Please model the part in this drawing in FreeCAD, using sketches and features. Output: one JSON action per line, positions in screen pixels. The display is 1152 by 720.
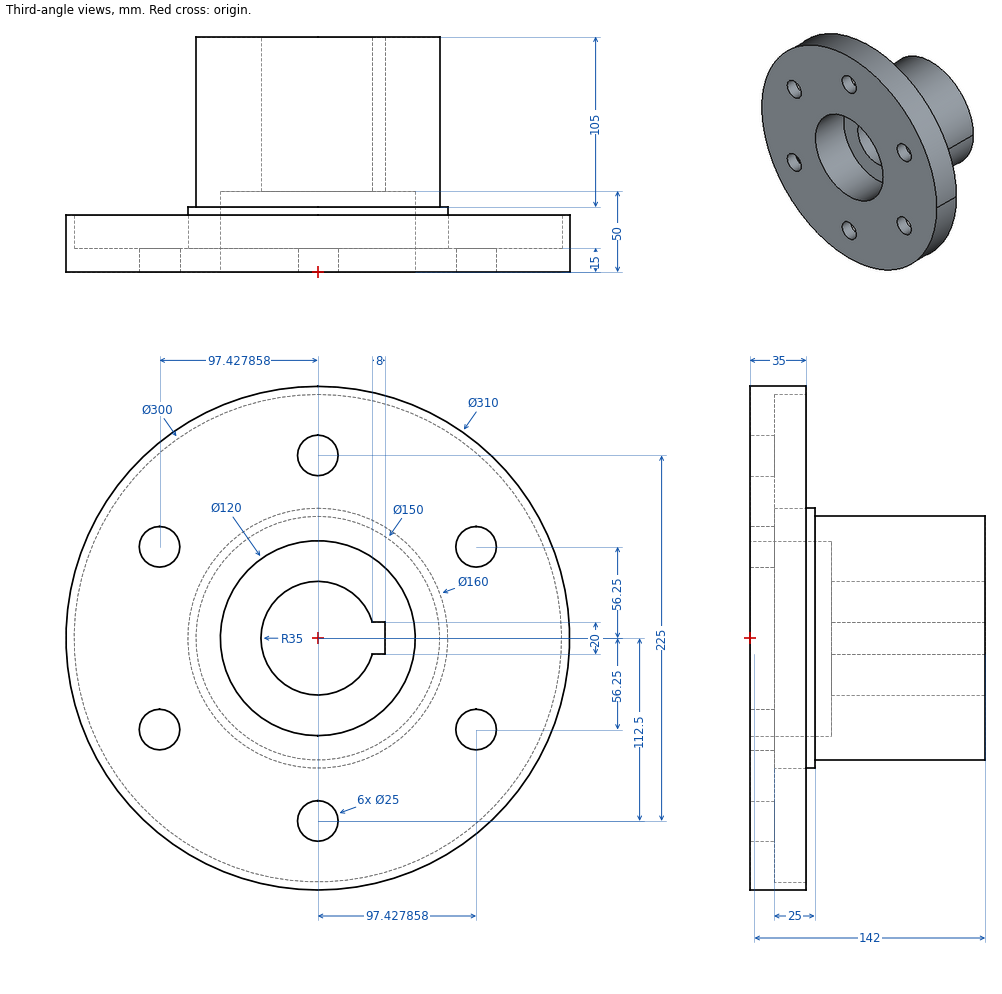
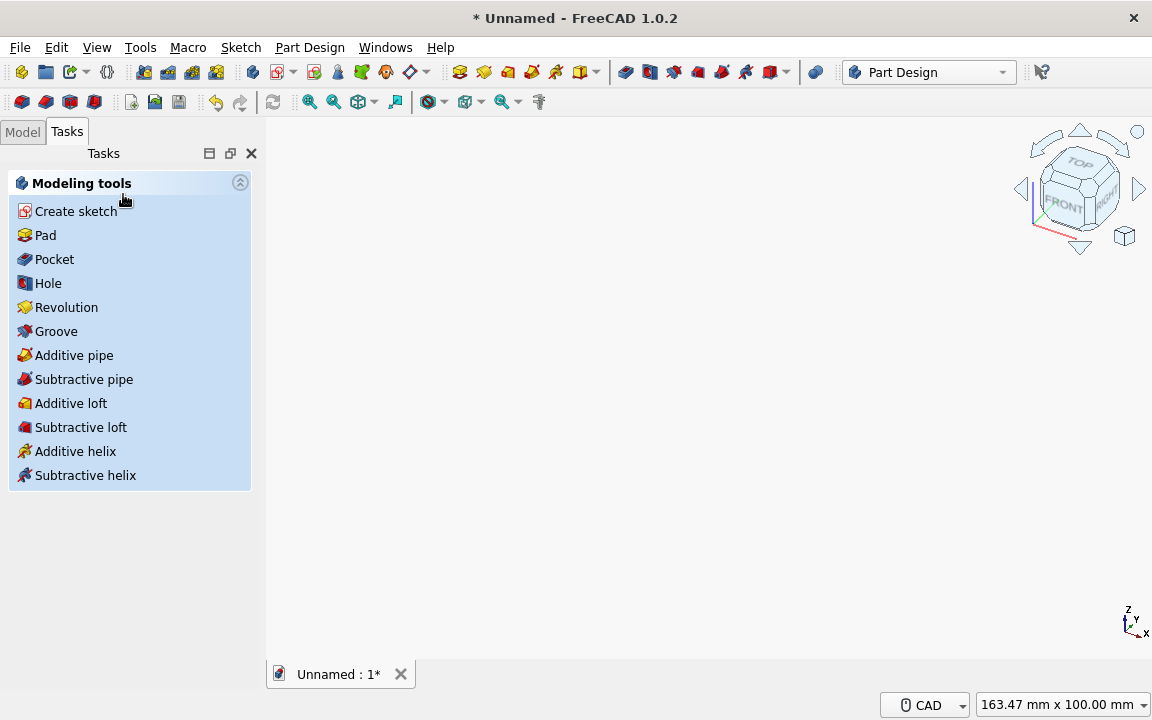
{"action": "left_click", "coordinate": [460, 72]}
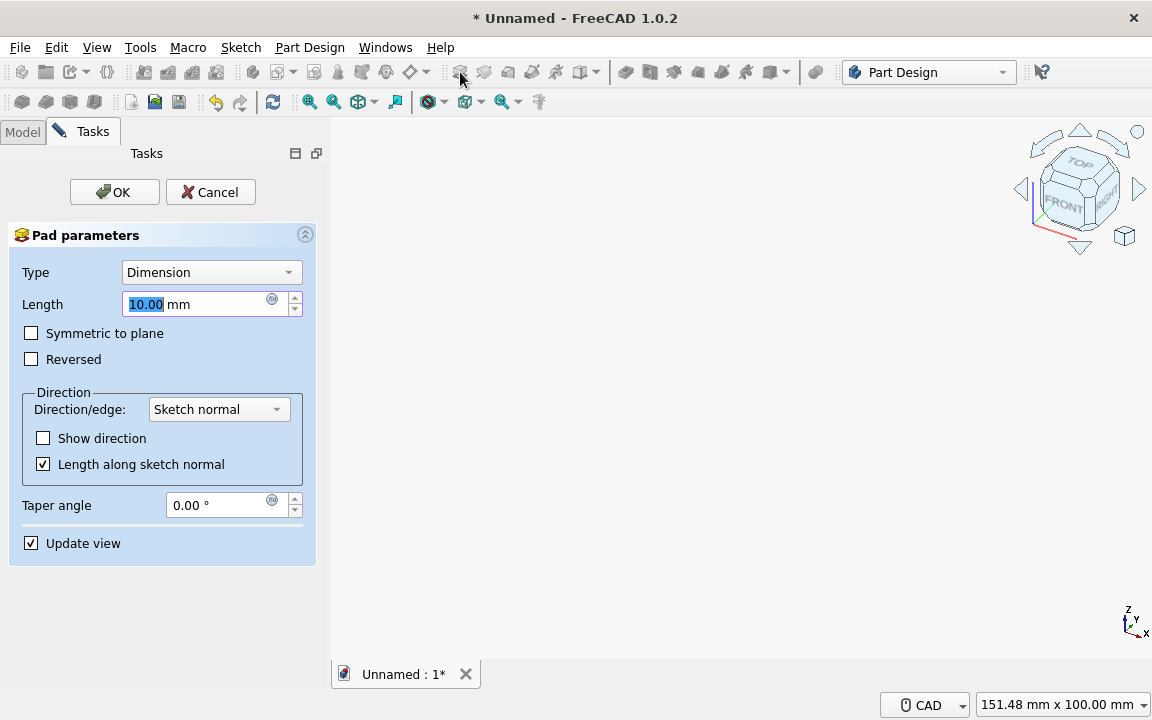
{"action": "type", "text": "35"}
{"action": "key", "text": "Tab"}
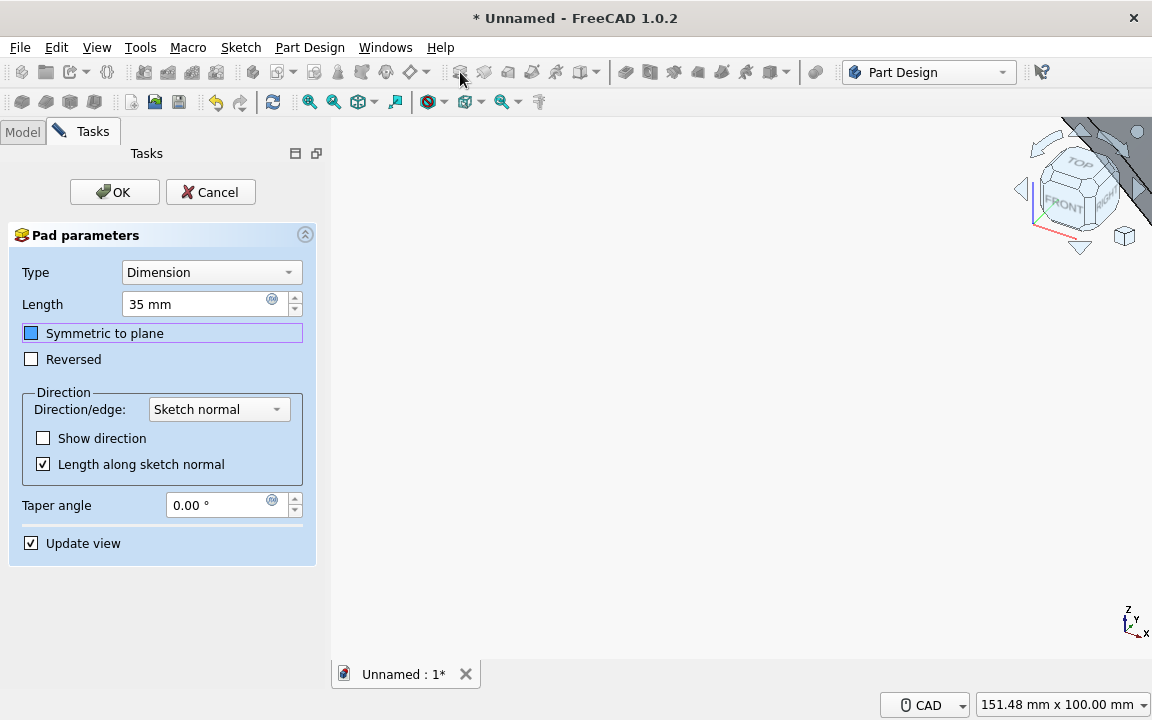
{"action": "left_click", "coordinate": [30, 359]}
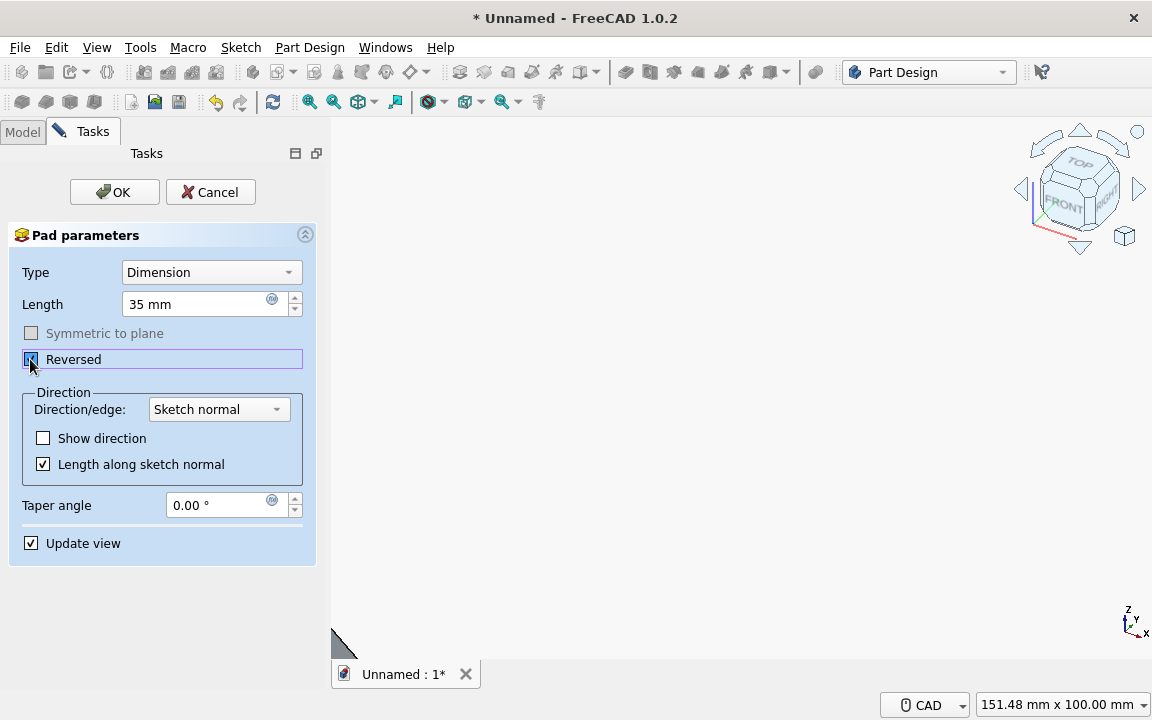
{"action": "left_click", "coordinate": [115, 192]}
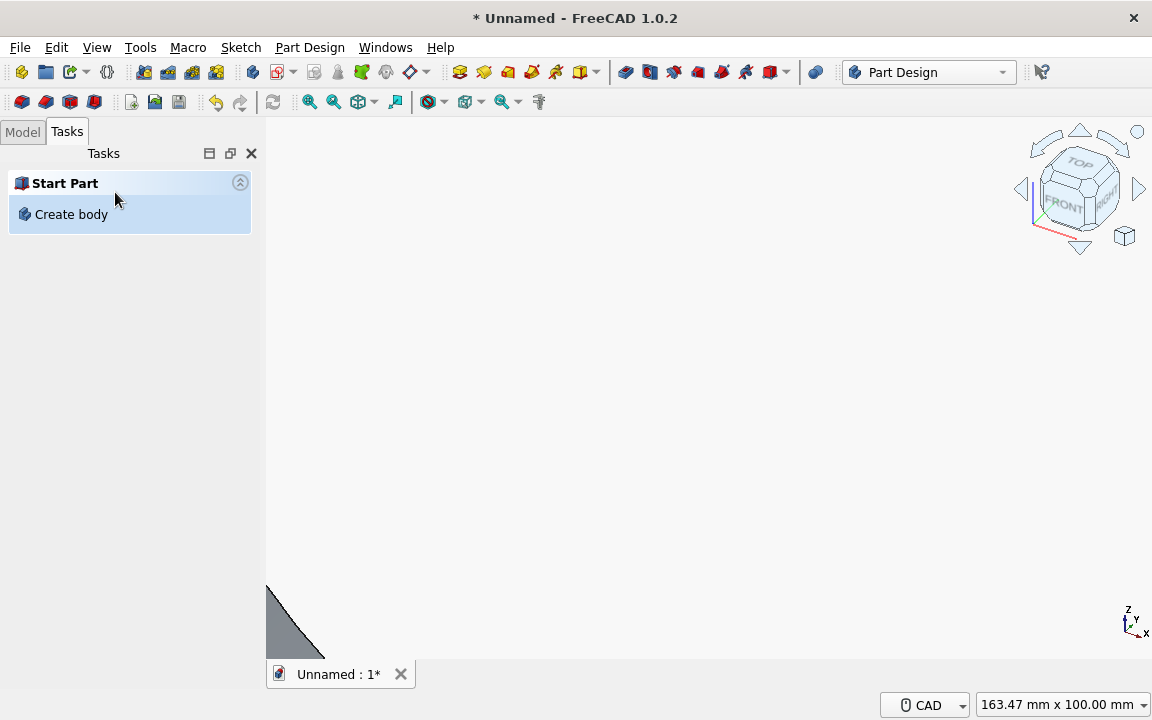
{"action": "left_click", "coordinate": [310, 102]}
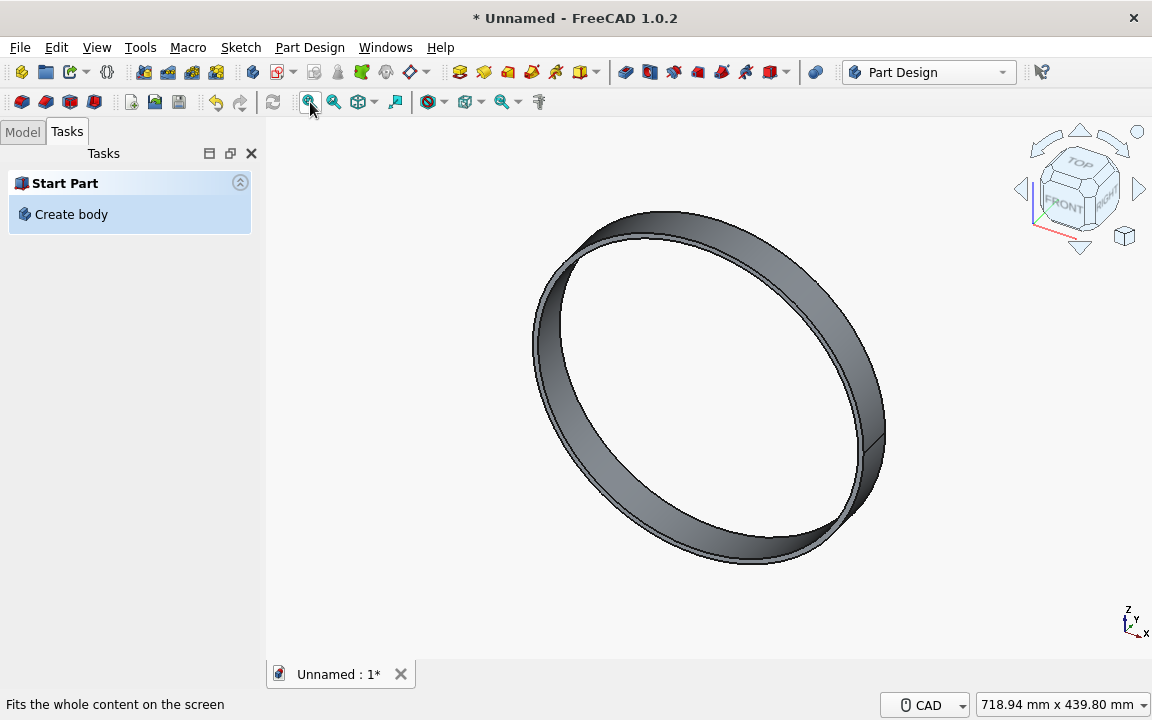
{"action": "left_click", "coordinate": [278, 72]}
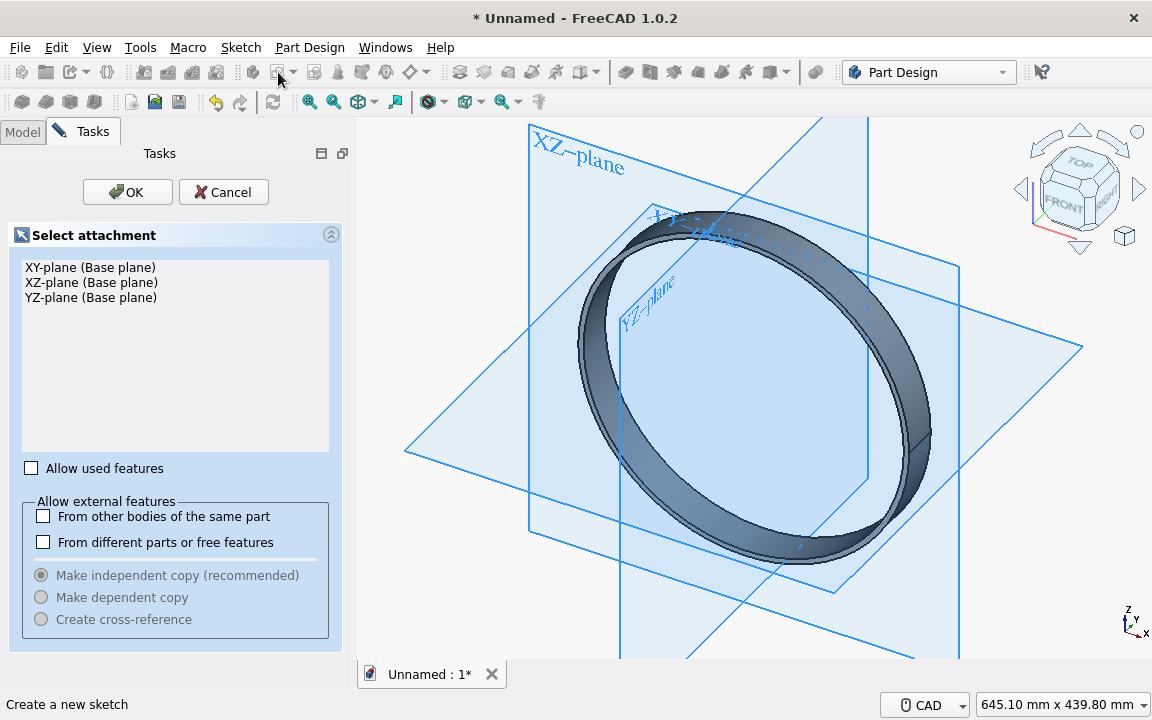
{"action": "left_click", "coordinate": [82, 282]}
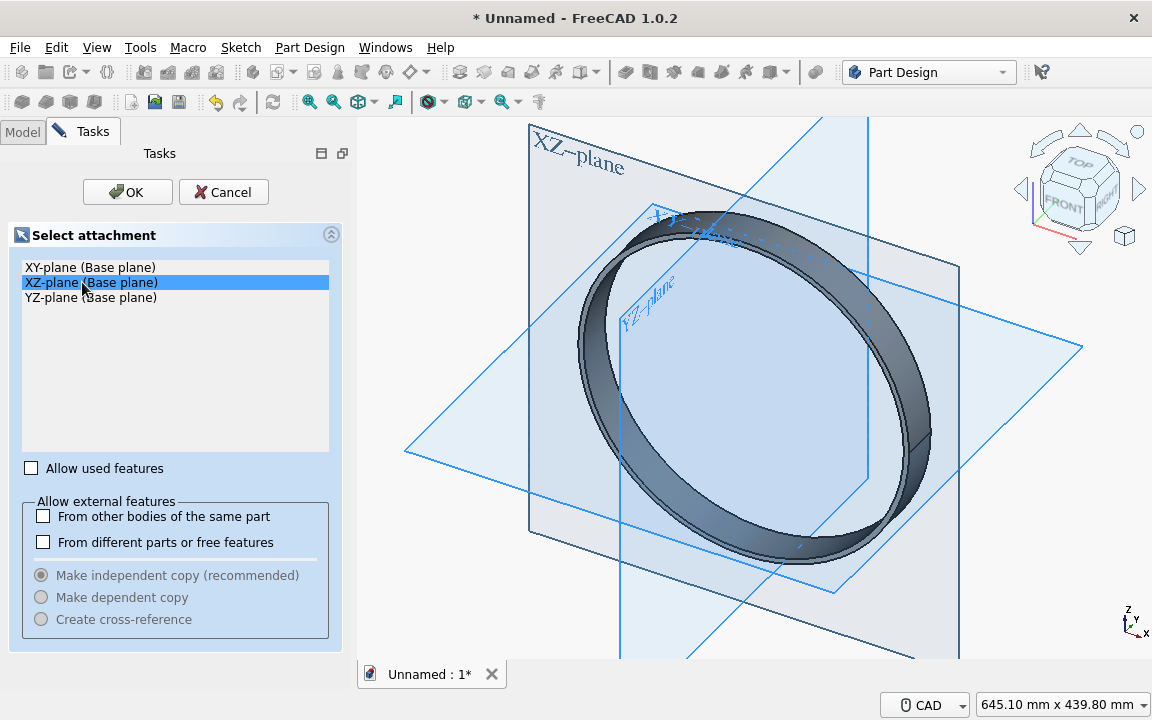
{"action": "left_click", "coordinate": [128, 192]}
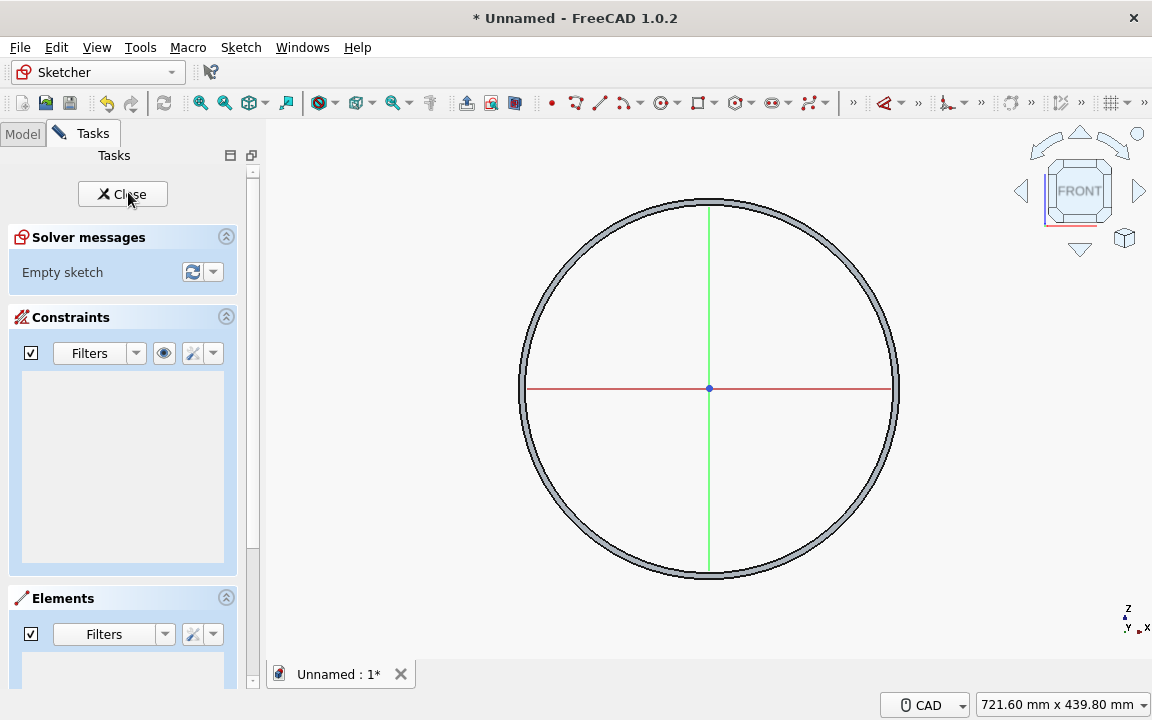
{"action": "left_click", "coordinate": [662, 104]}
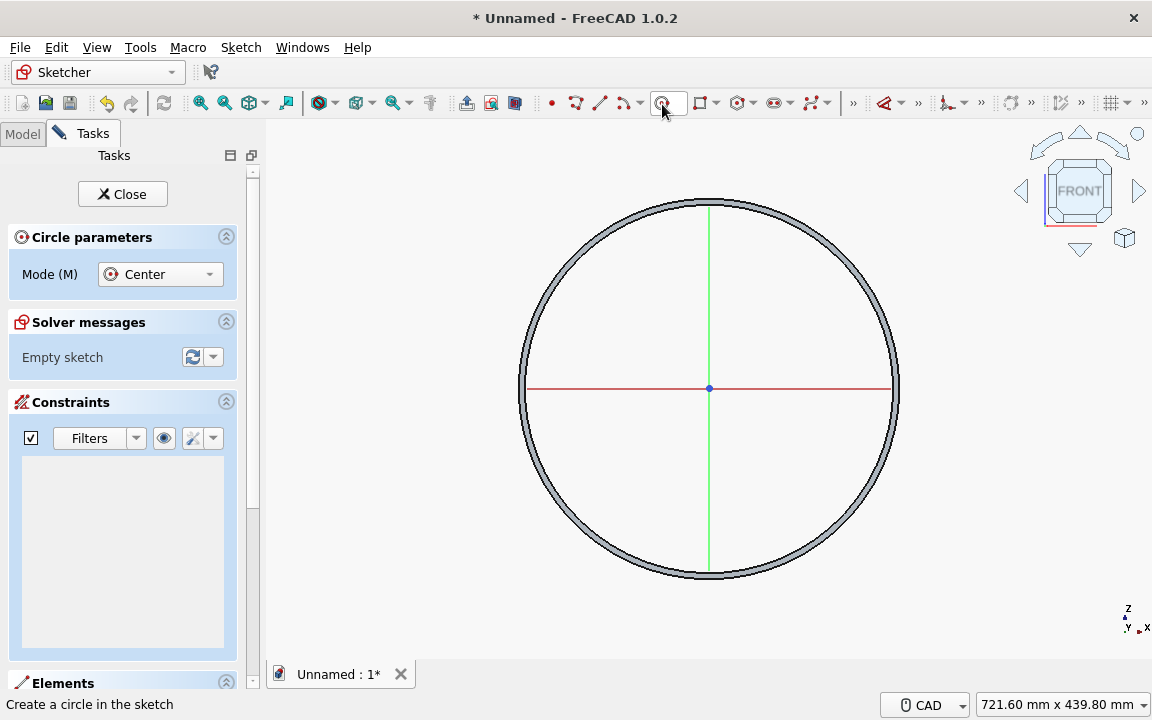
{"action": "left_click", "coordinate": [709, 389]}
{"action": "mouse_move", "coordinate": [839, 259]}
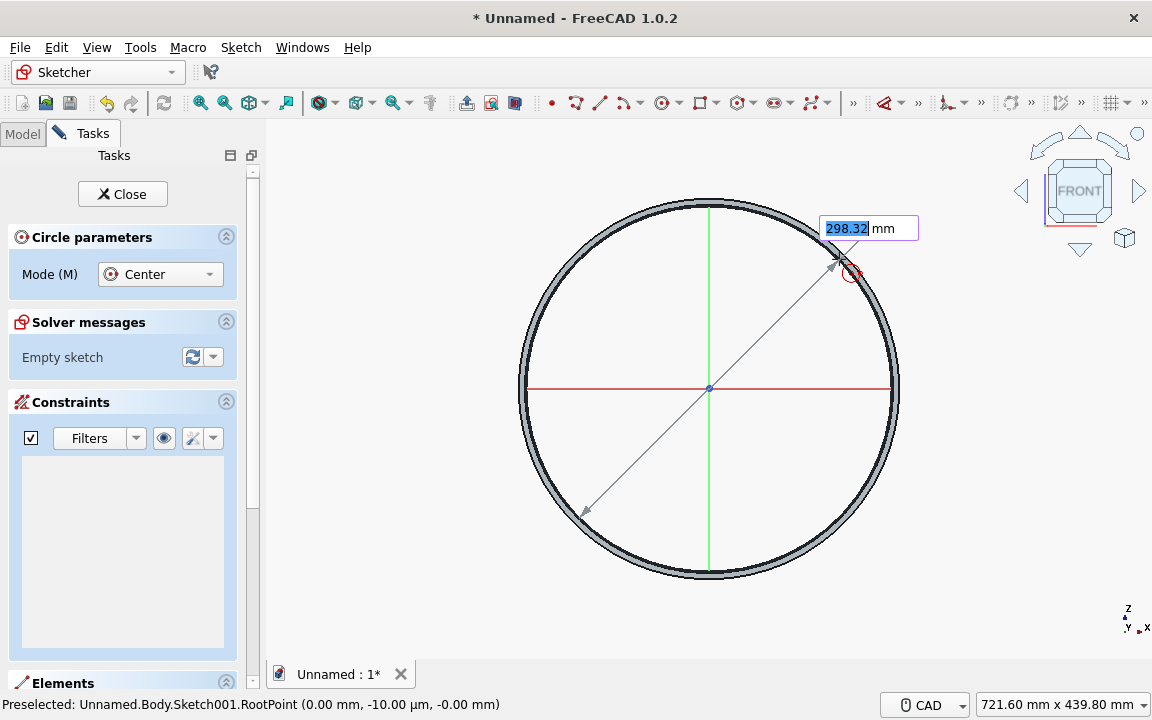
{"action": "type", "text": "300"}
{"action": "key", "text": "Return"}
{"action": "key", "text": "Escape"}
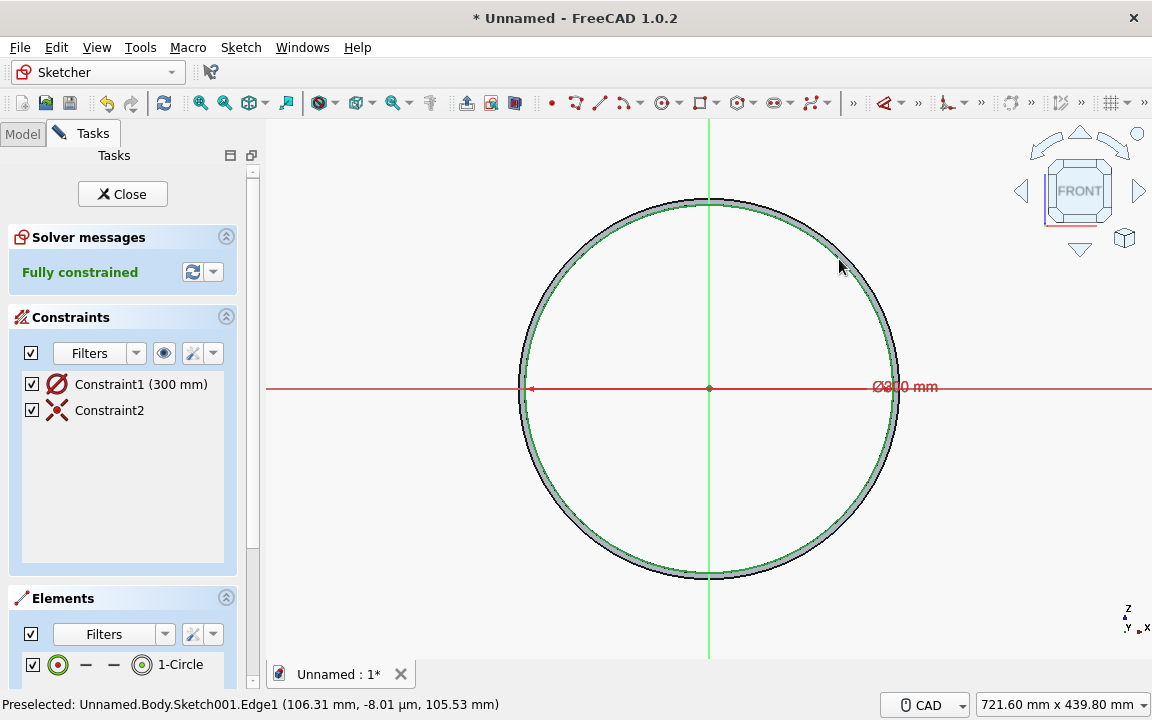
{"action": "left_click", "coordinate": [123, 194]}